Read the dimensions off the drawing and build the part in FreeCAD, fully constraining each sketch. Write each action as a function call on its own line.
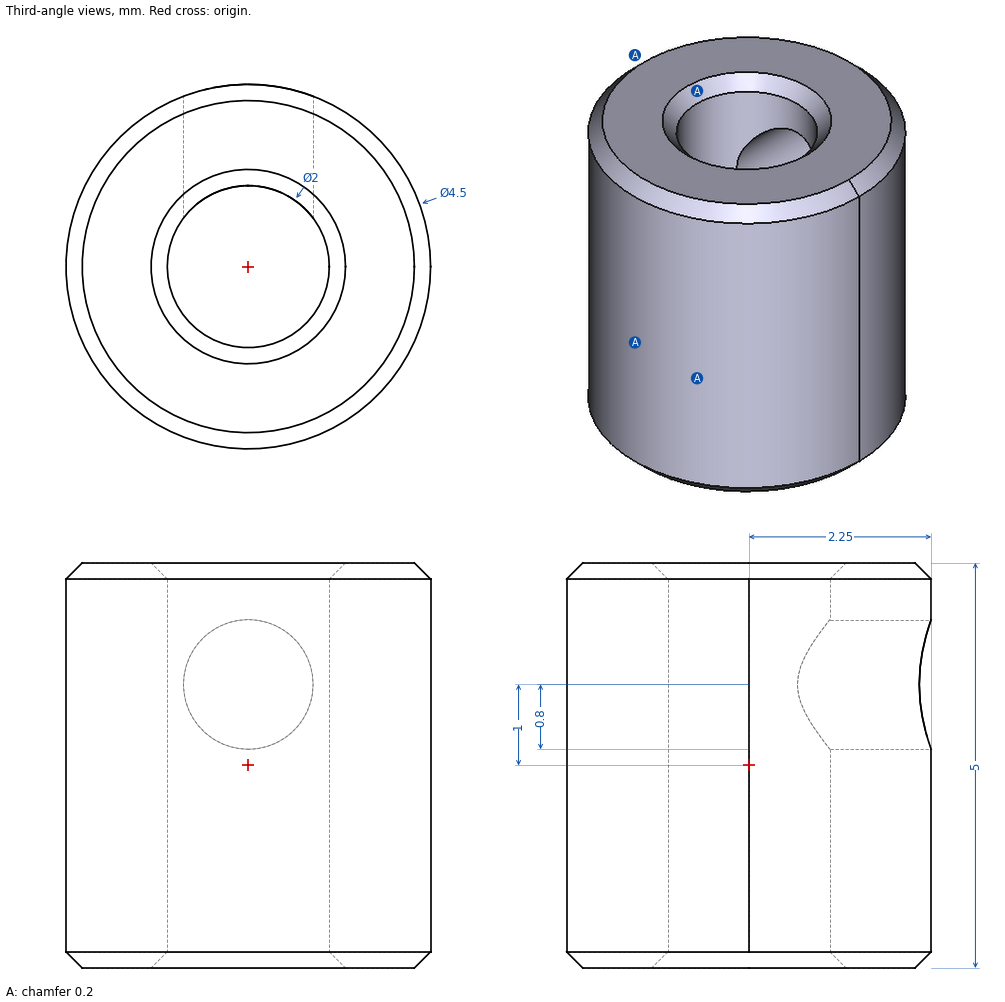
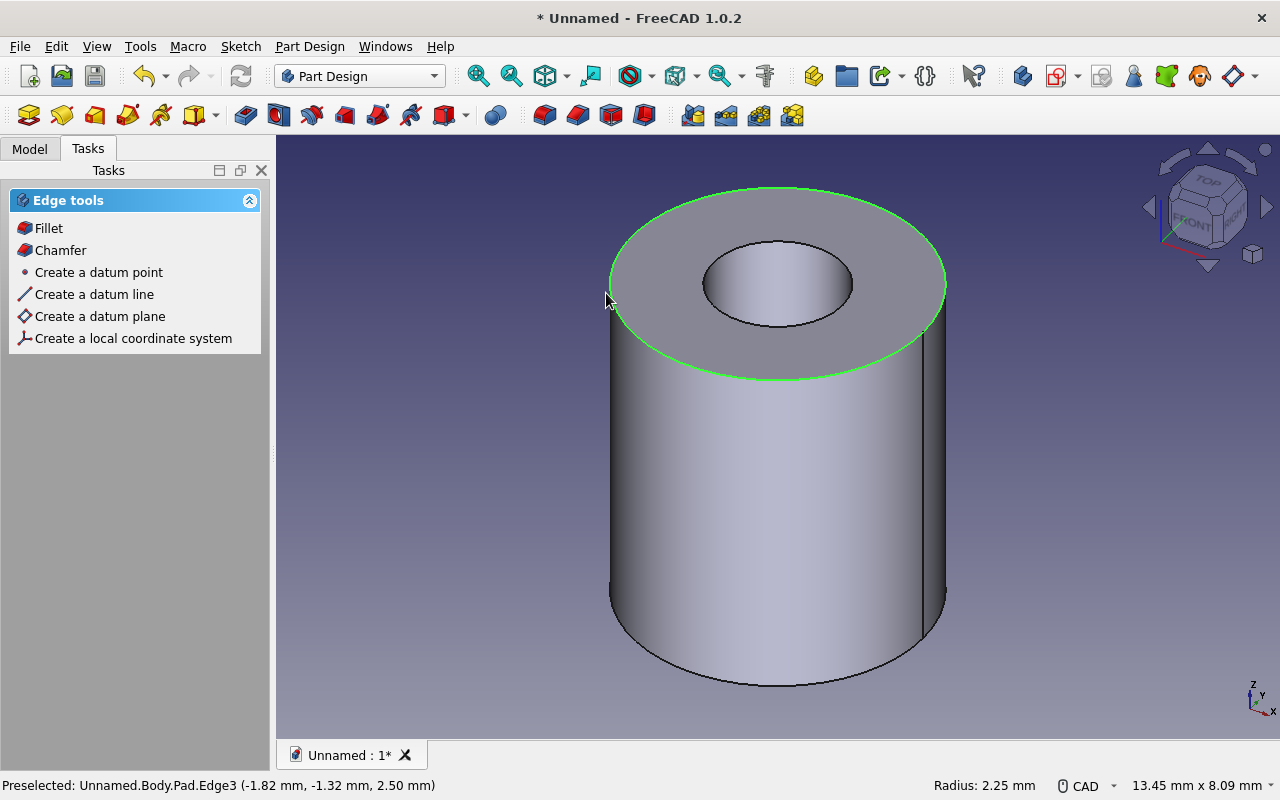
click(713, 262, ctrl)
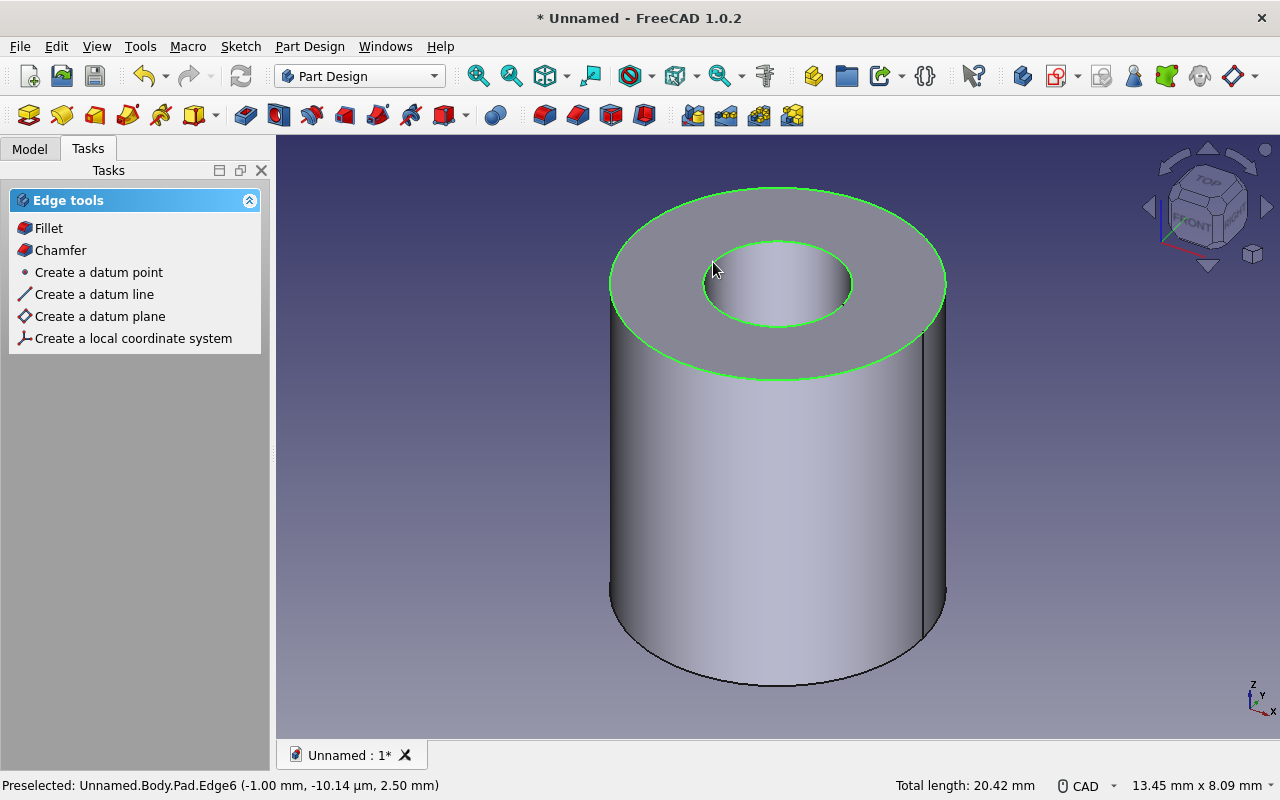
key(0)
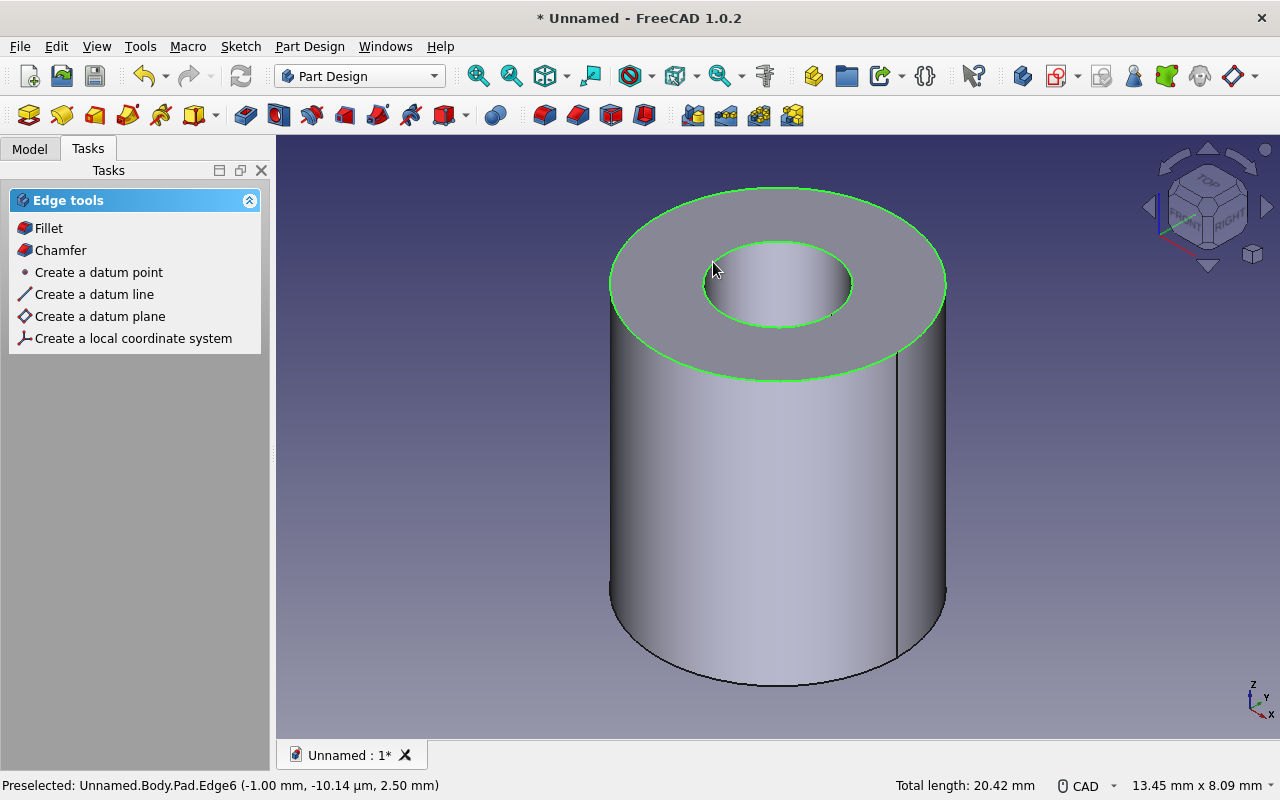
key(2)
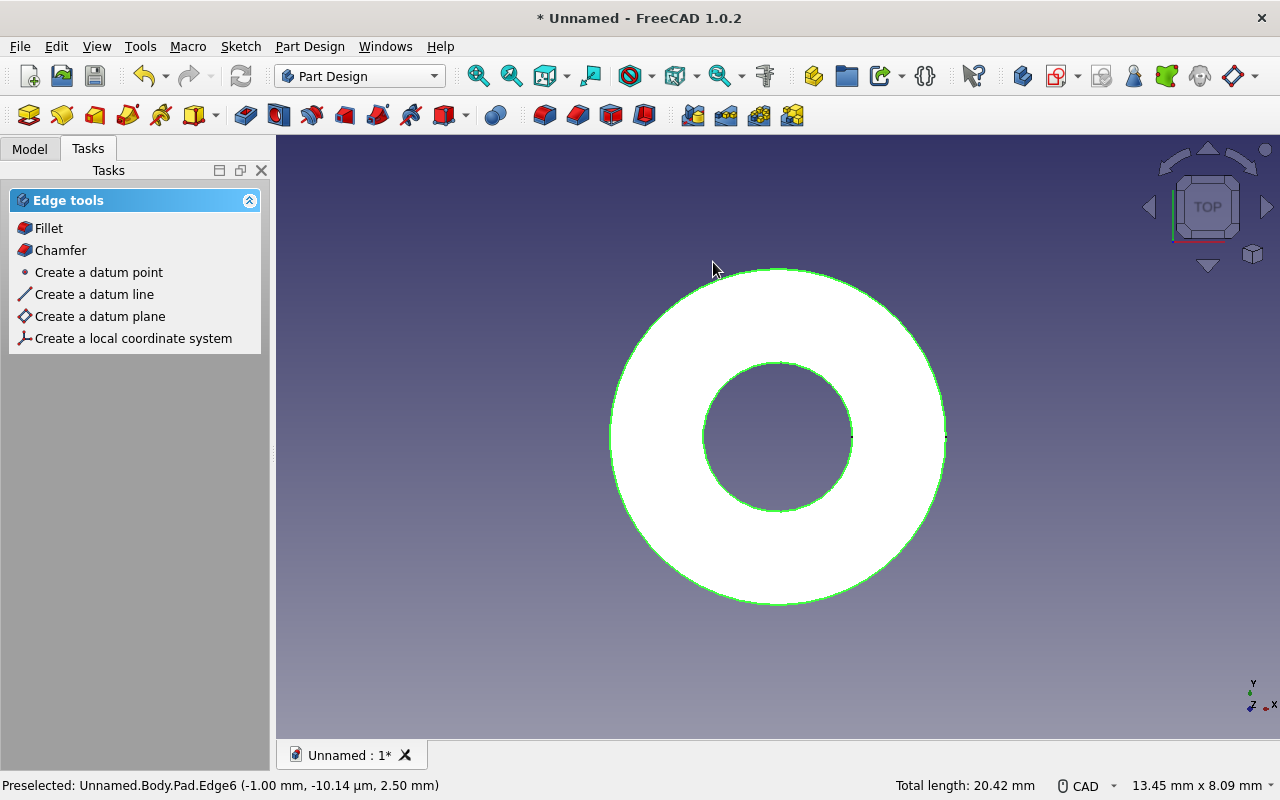
key(1)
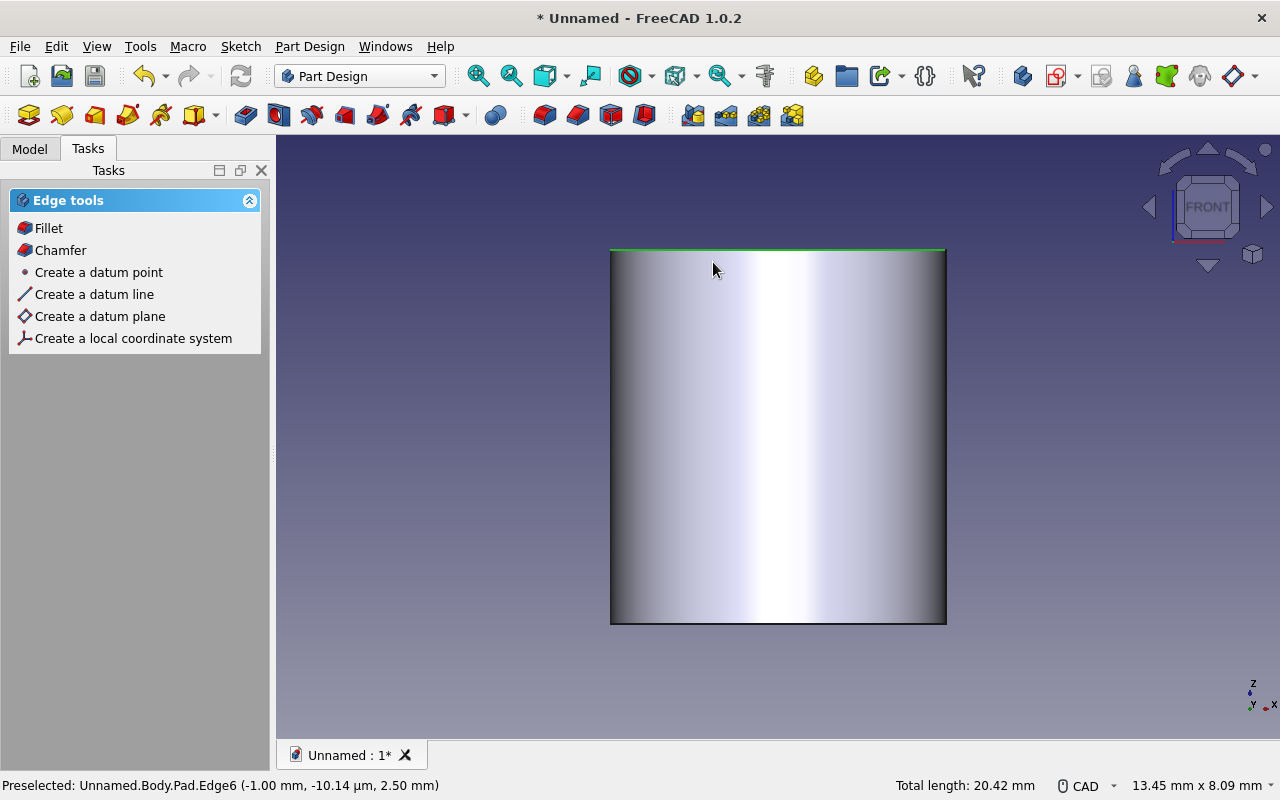
click(642, 623, ctrl)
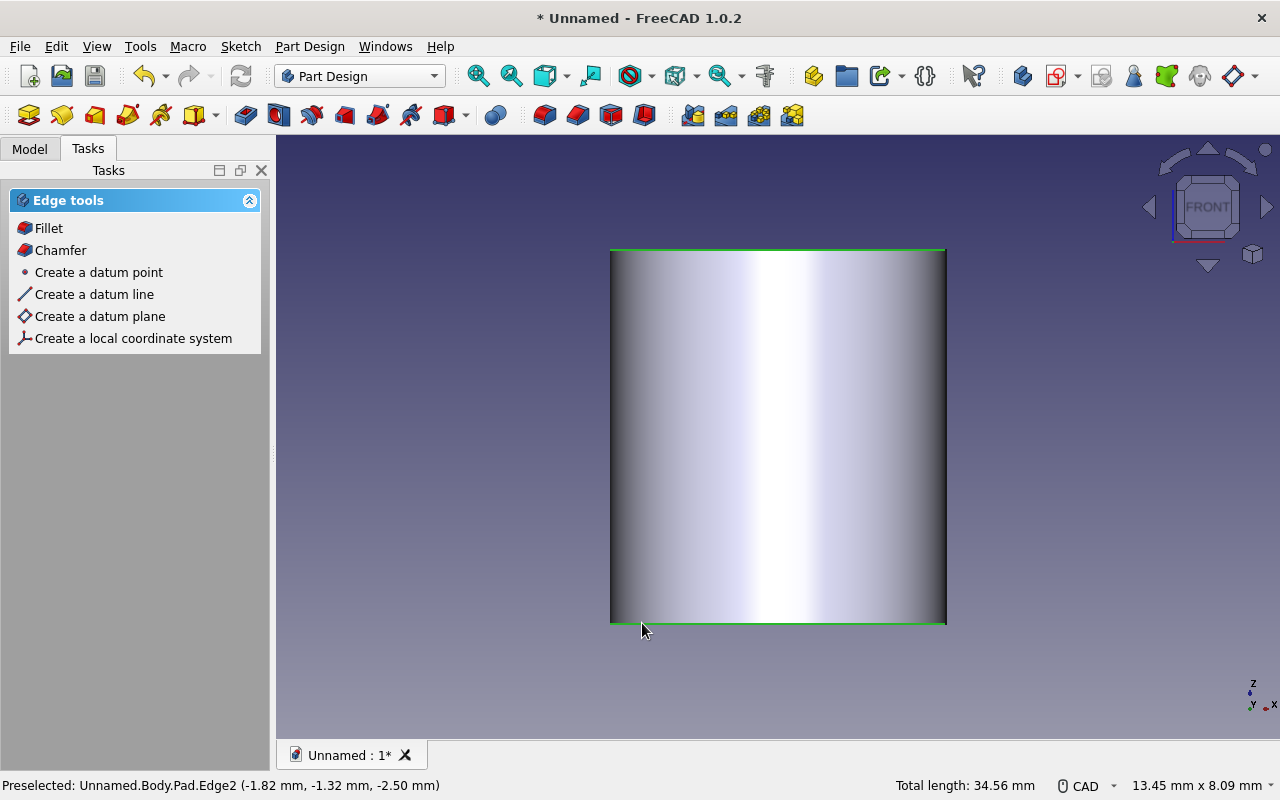
key(3)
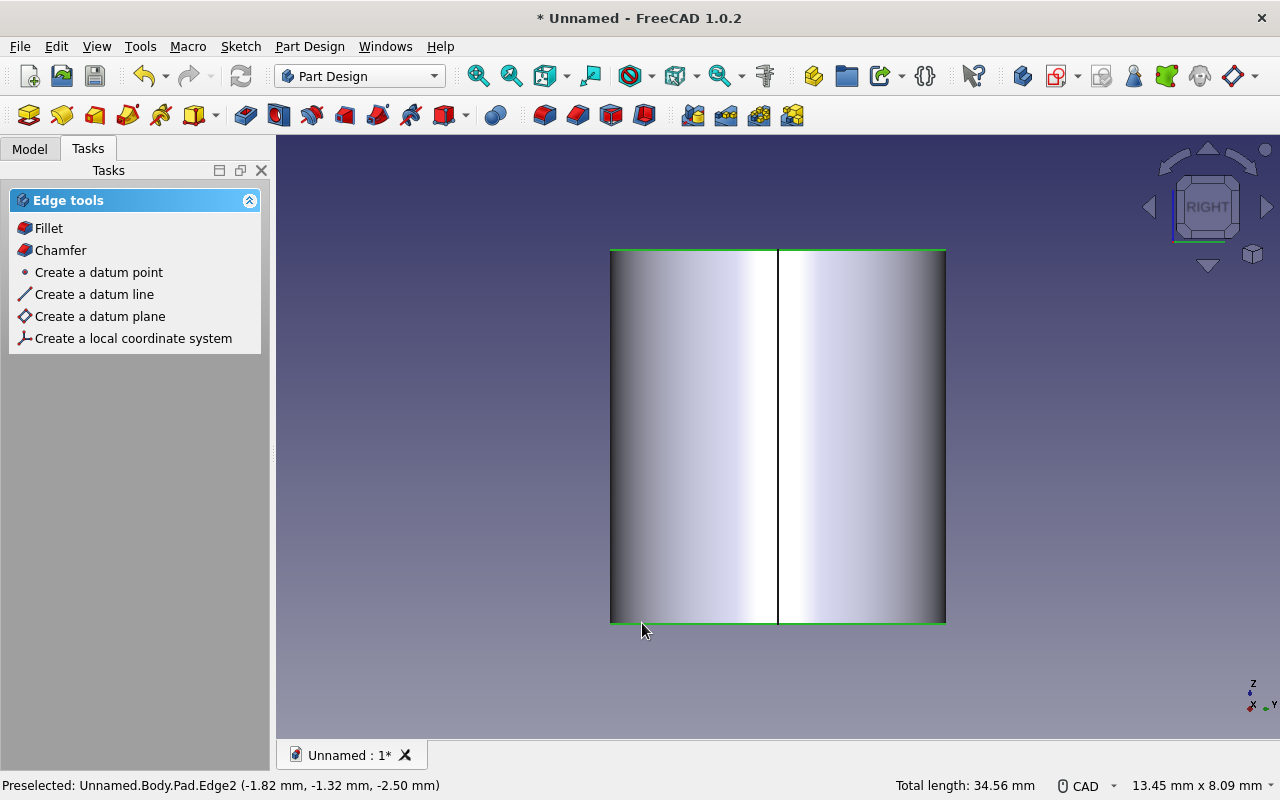
key(5)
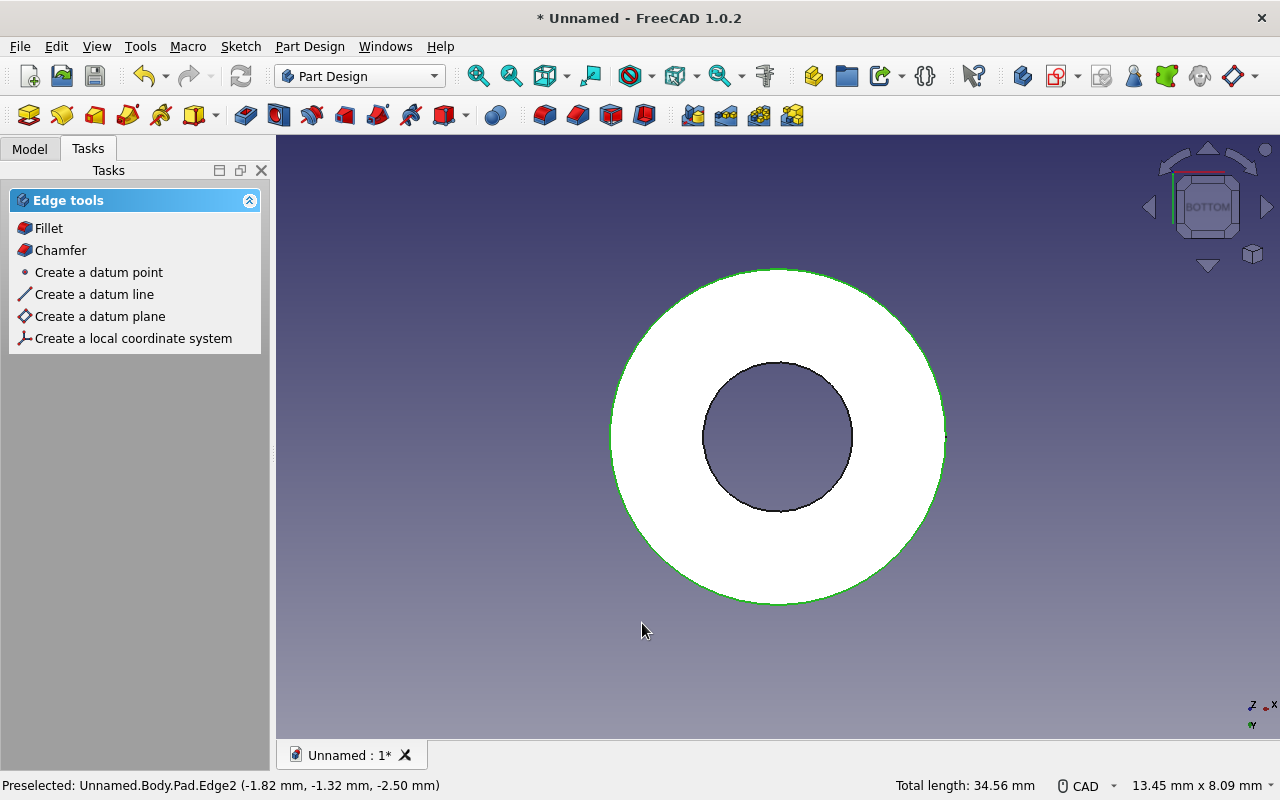
click(703, 436, ctrl)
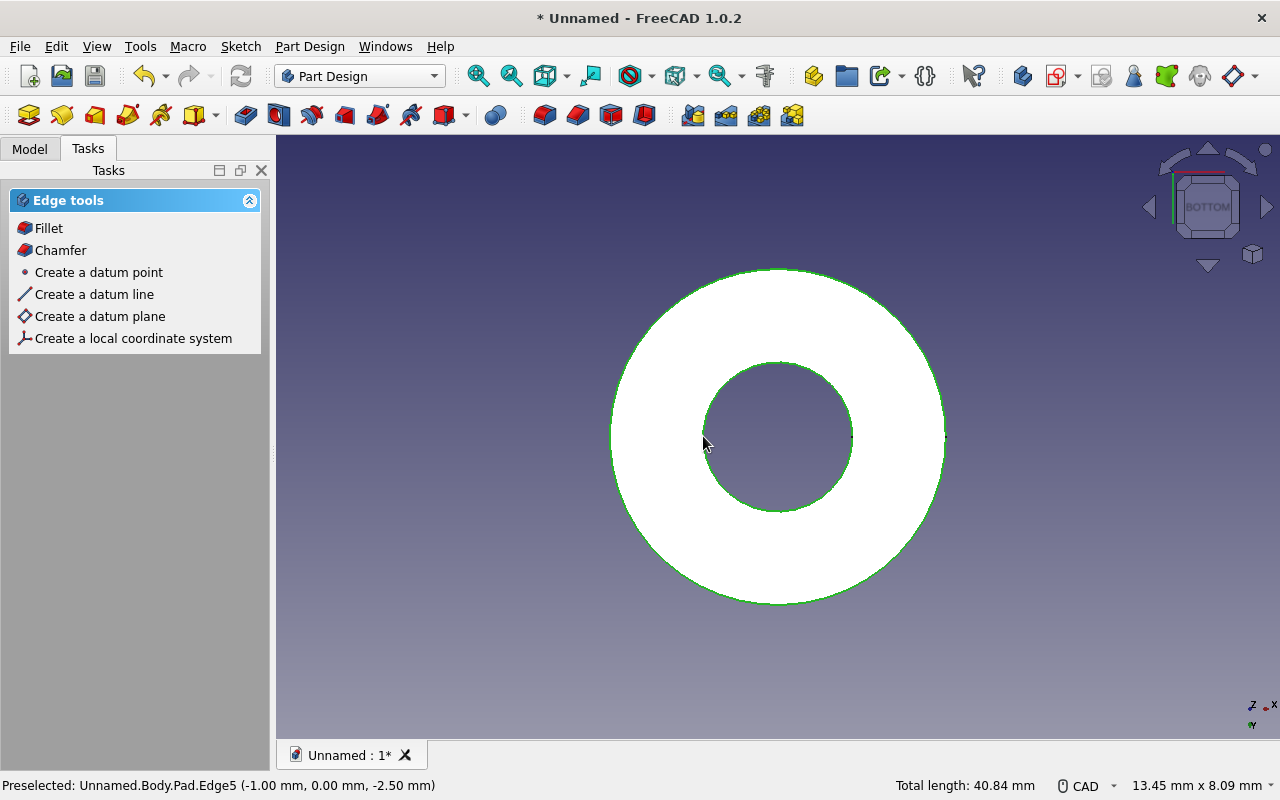
click(578, 116)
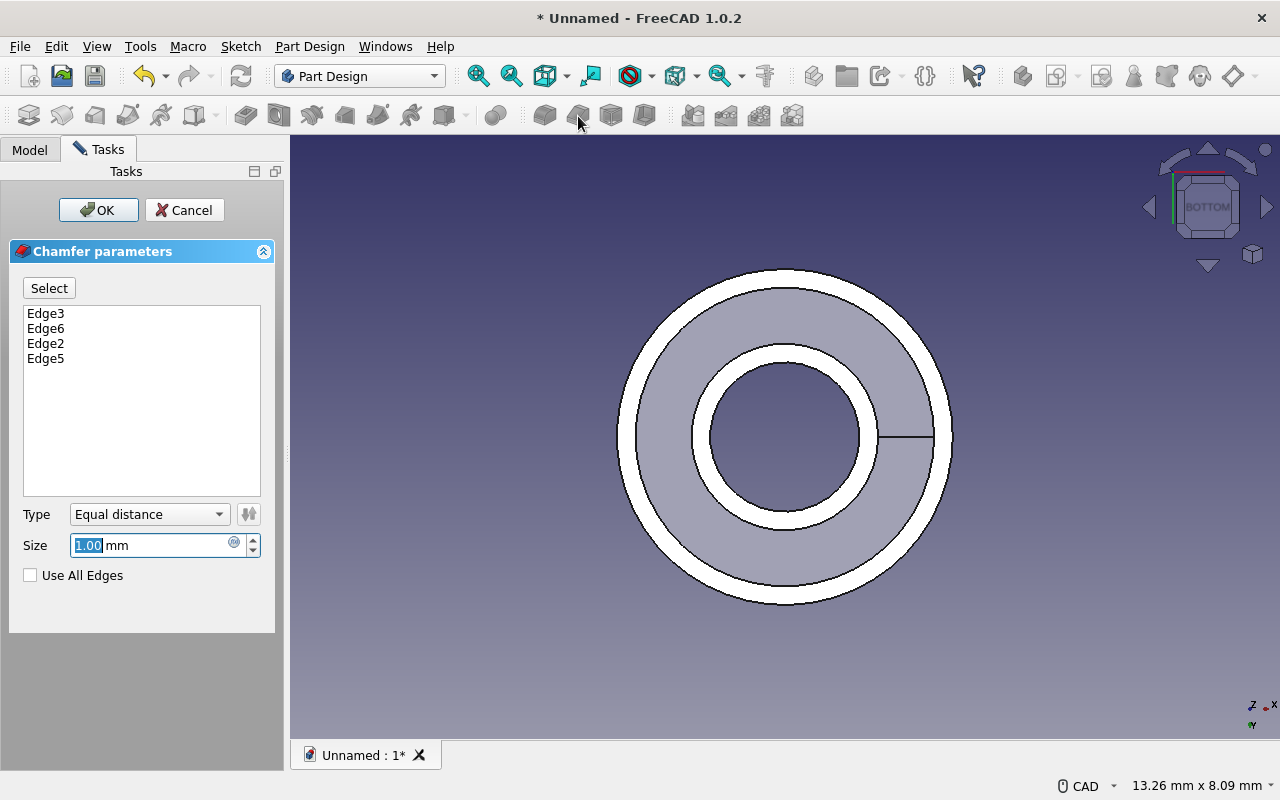
text(0.2)
key(Tab)